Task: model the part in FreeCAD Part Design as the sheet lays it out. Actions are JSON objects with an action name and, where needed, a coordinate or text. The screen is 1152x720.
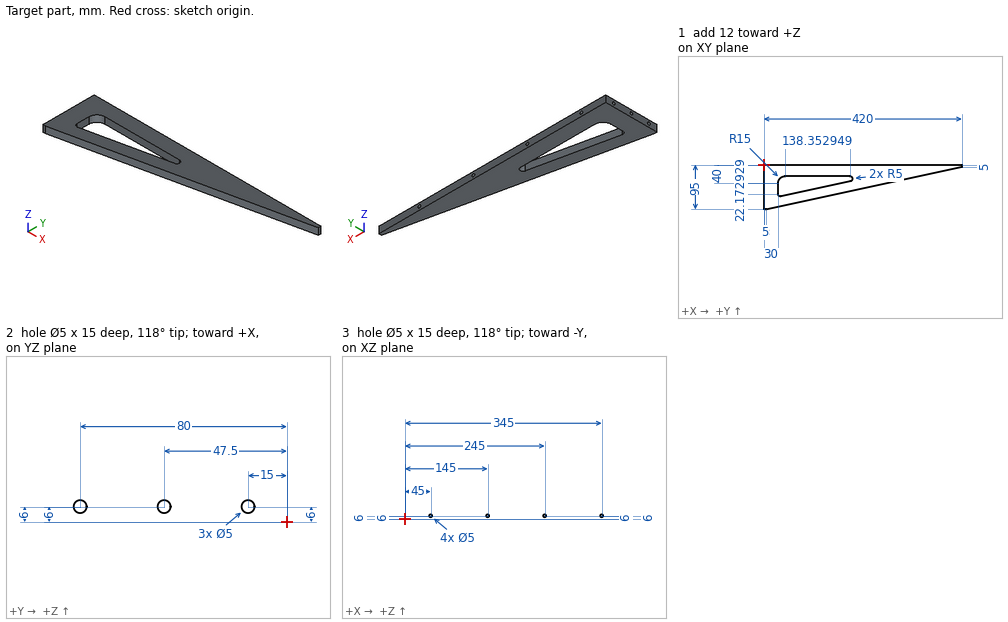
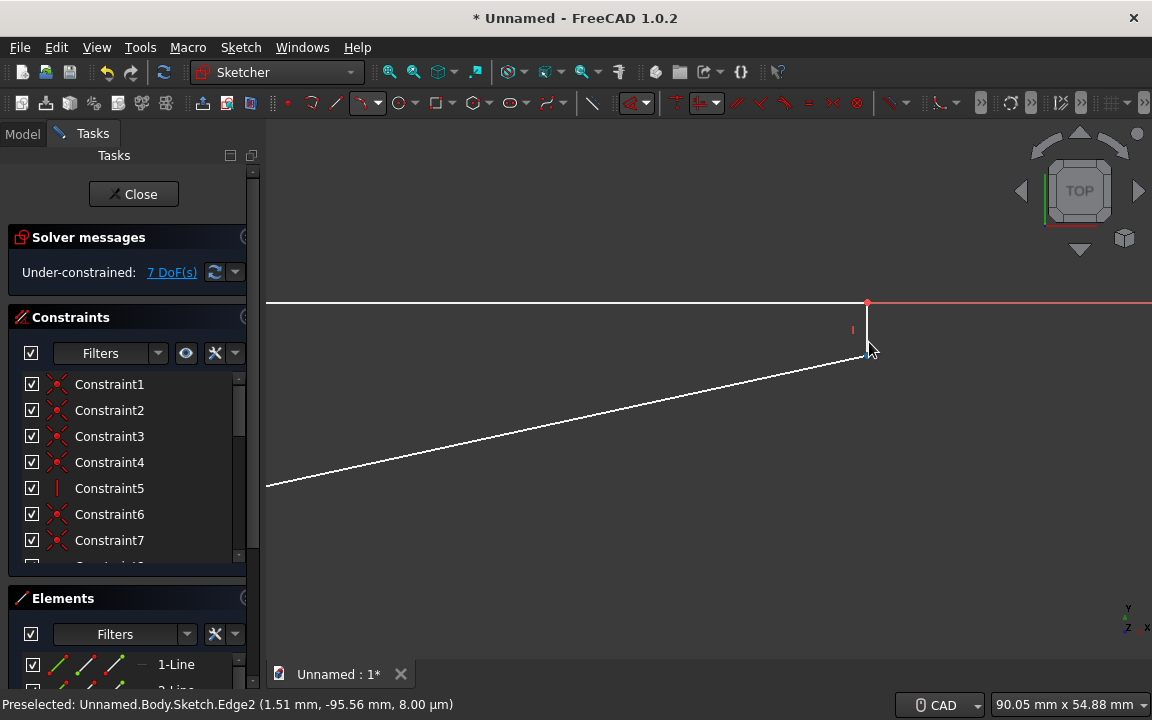
{"action": "left_click", "coordinate": [867, 340]}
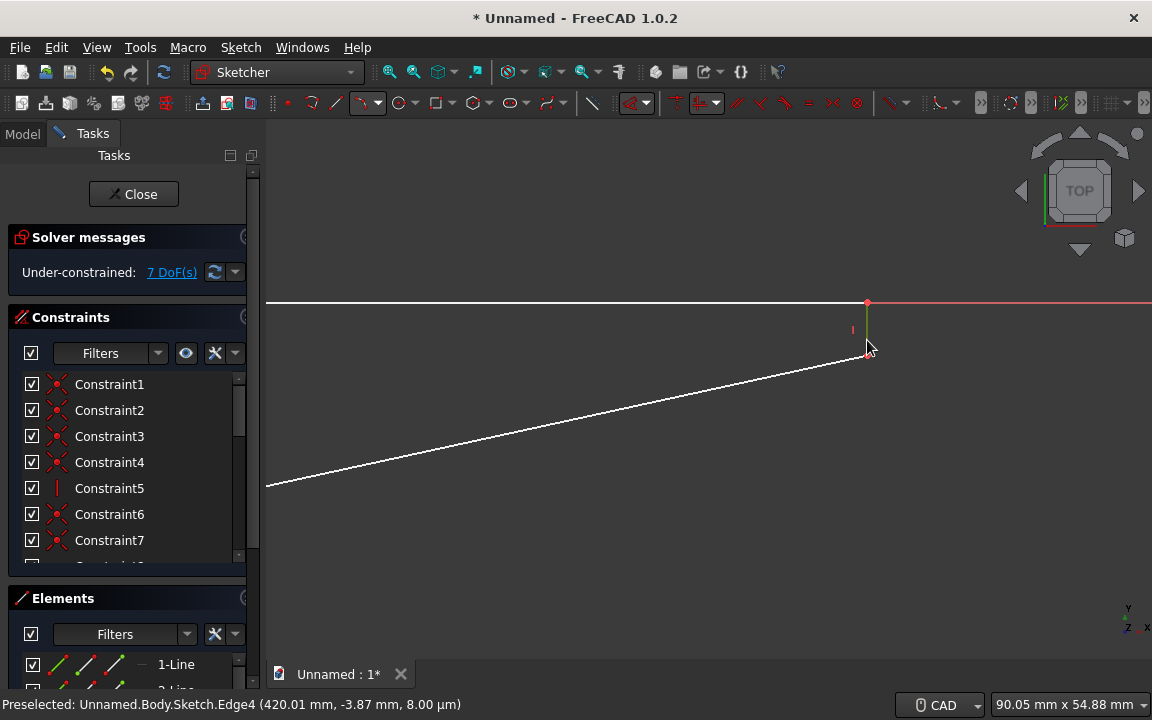
{"action": "left_click", "coordinate": [648, 104]}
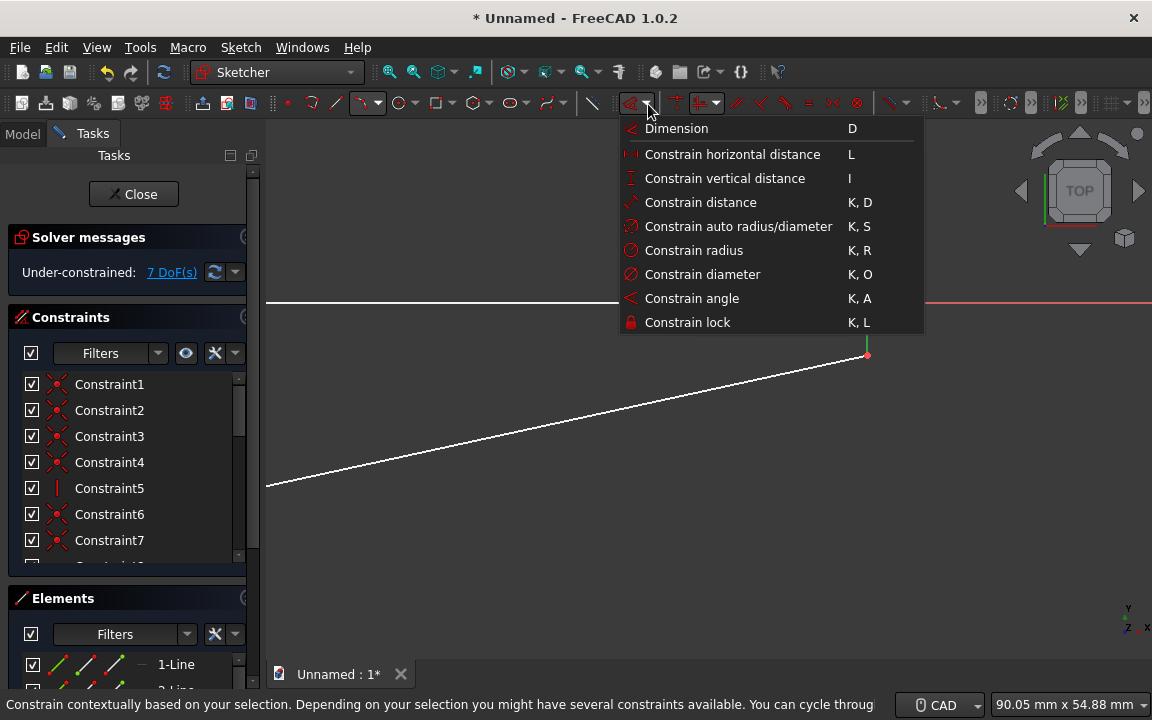
{"action": "left_click", "coordinate": [772, 178]}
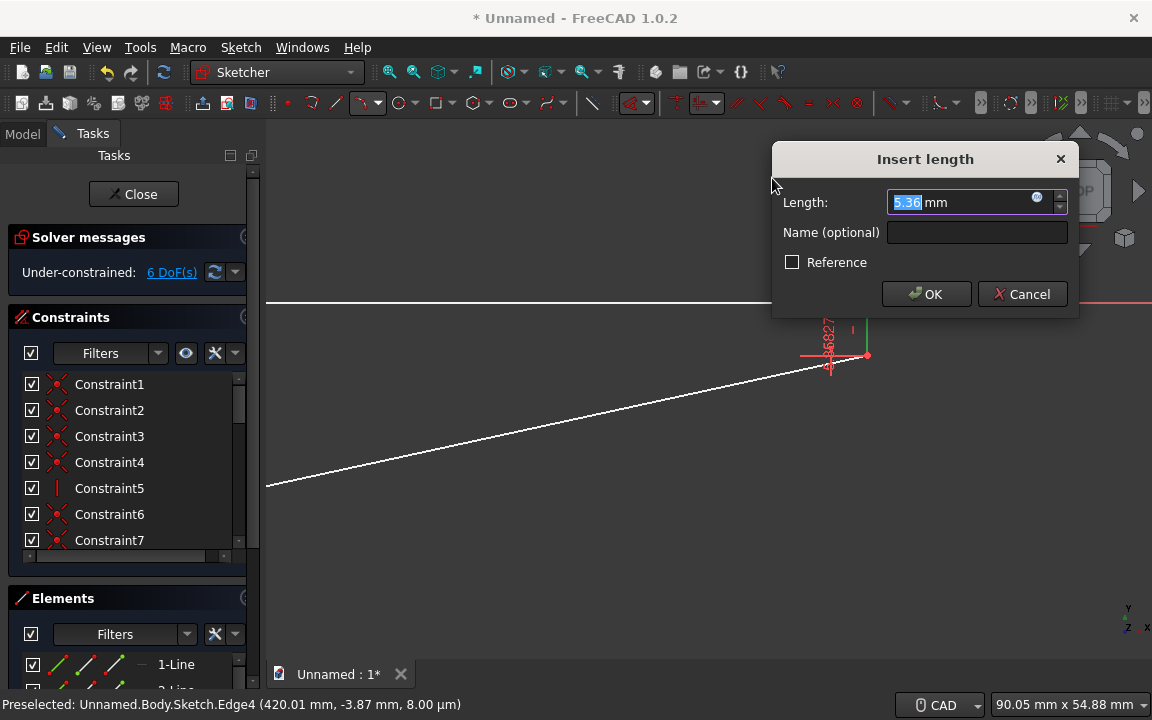
{"action": "type", "text": "5"}
{"action": "key", "text": "Return"}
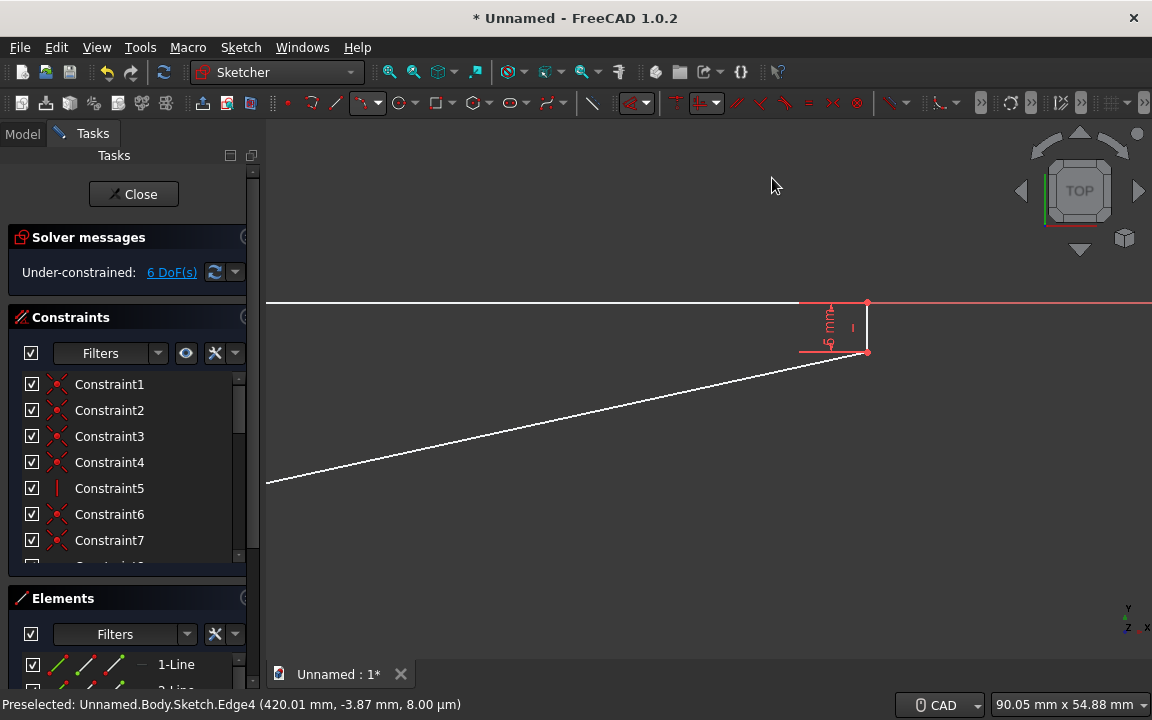
{"action": "scroll", "coordinate": [870, 341], "scroll_direction": "down", "scroll_amount": 11}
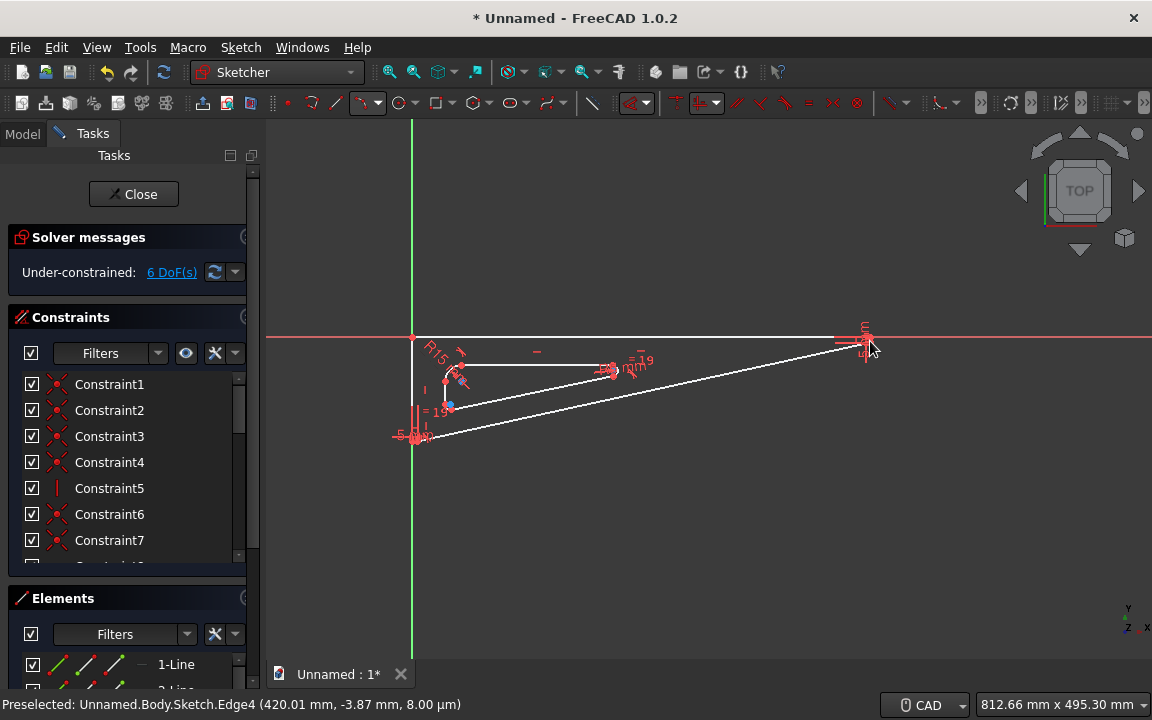
{"action": "left_click", "coordinate": [412, 368]}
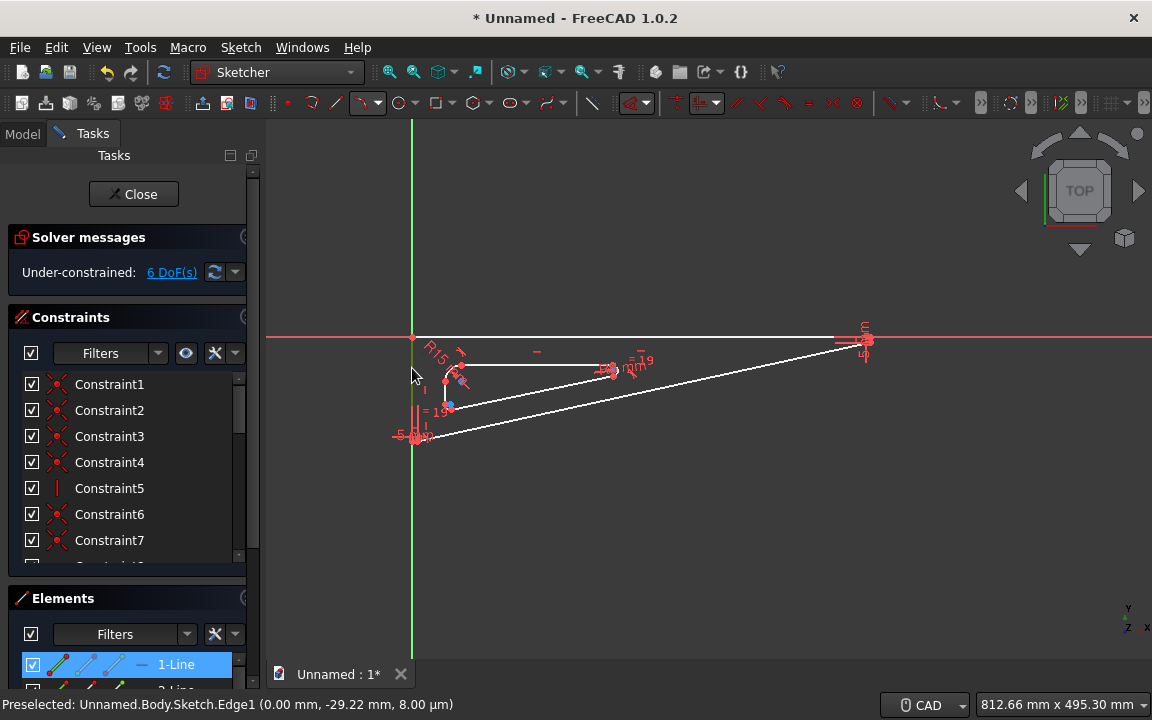
{"action": "key", "text": "i"}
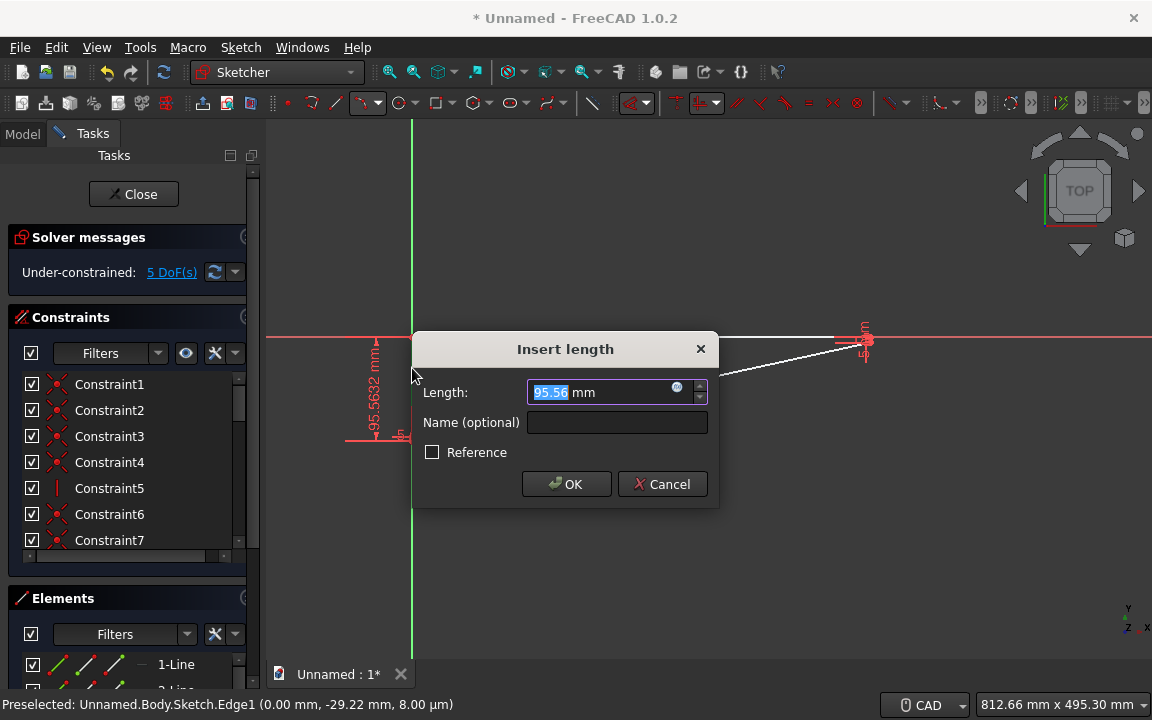
{"action": "type", "text": "95"}
{"action": "key", "text": "Return"}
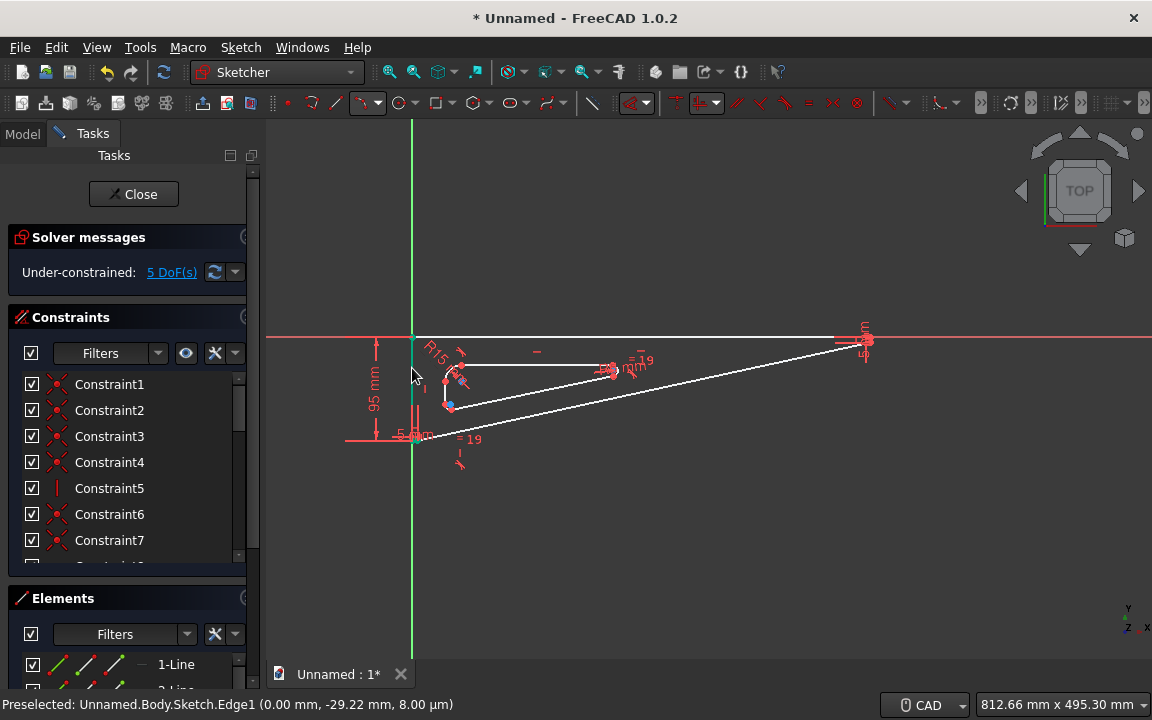
{"action": "left_click", "coordinate": [733, 337]}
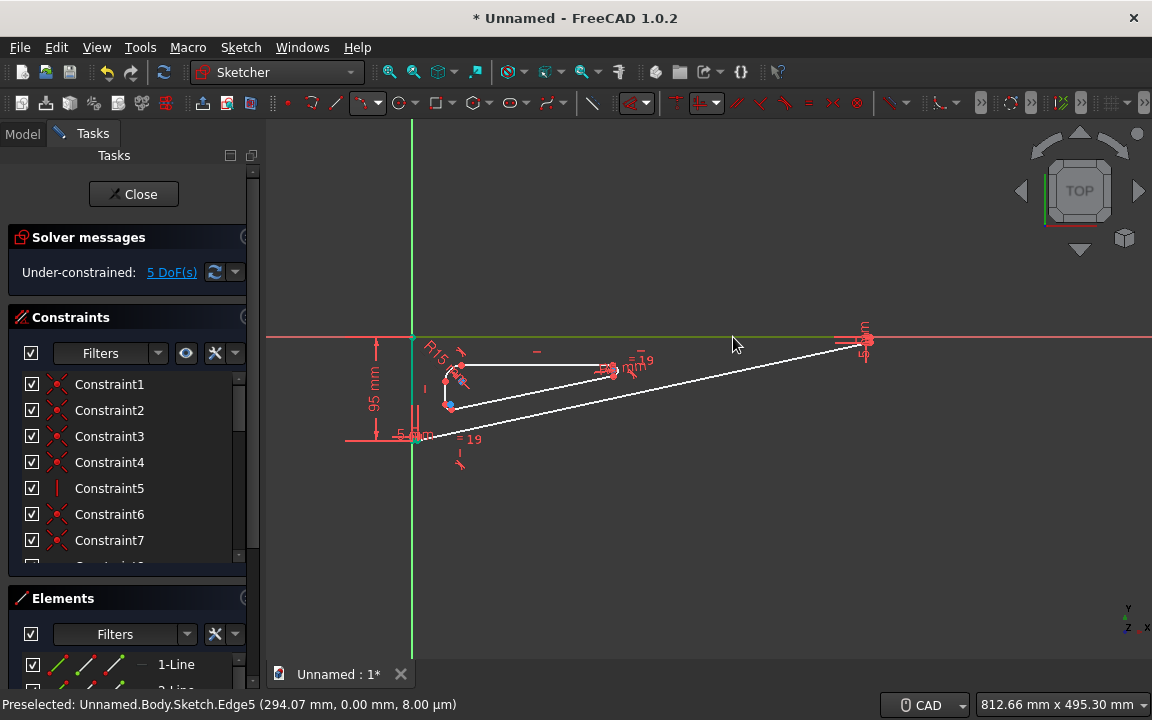
{"action": "left_click", "coordinate": [648, 104]}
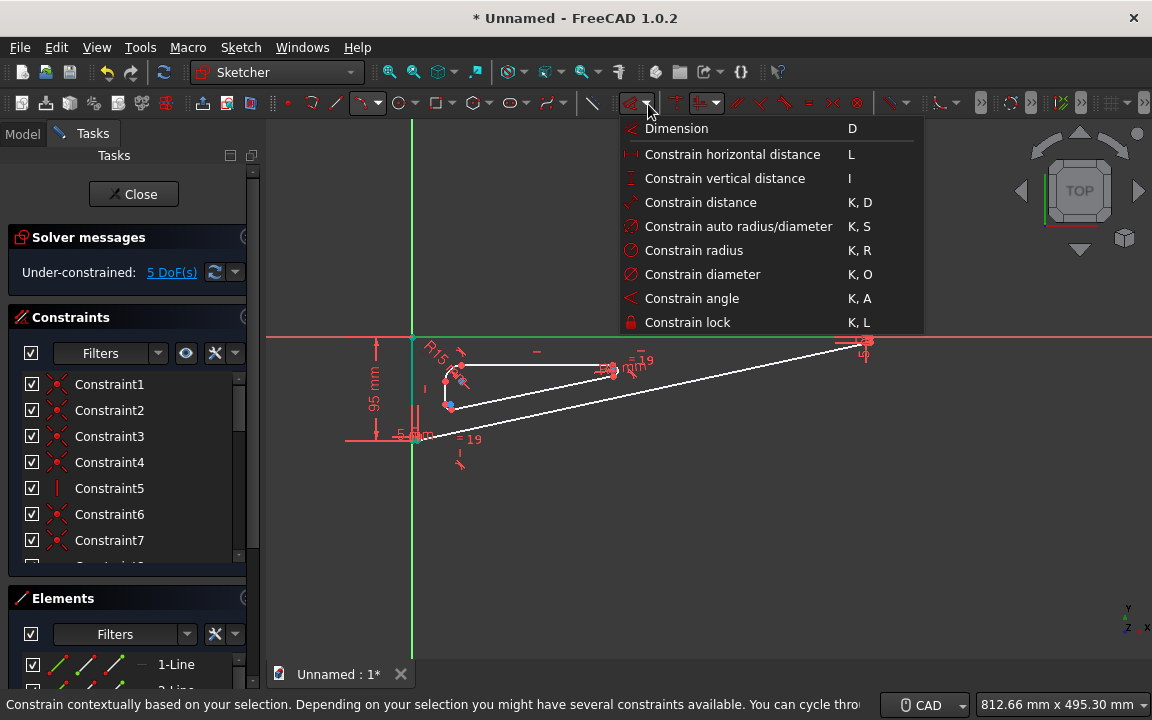
{"action": "left_click", "coordinate": [772, 154]}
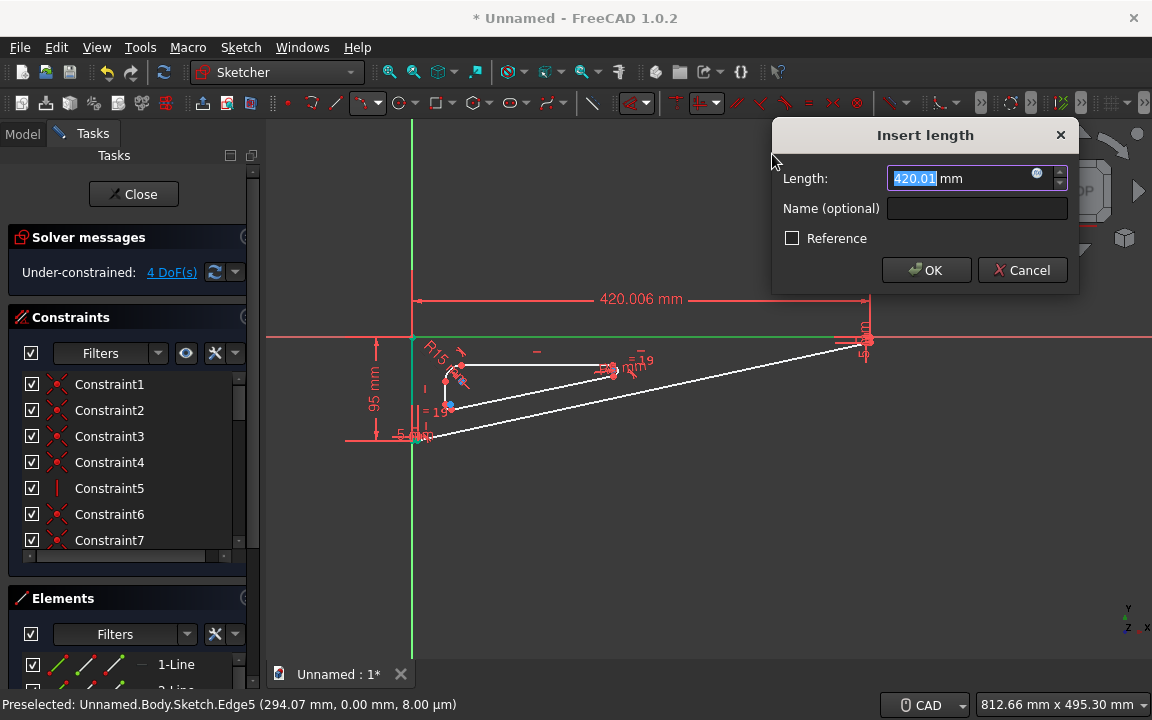
{"action": "type", "text": "420"}
{"action": "key", "text": "Return"}